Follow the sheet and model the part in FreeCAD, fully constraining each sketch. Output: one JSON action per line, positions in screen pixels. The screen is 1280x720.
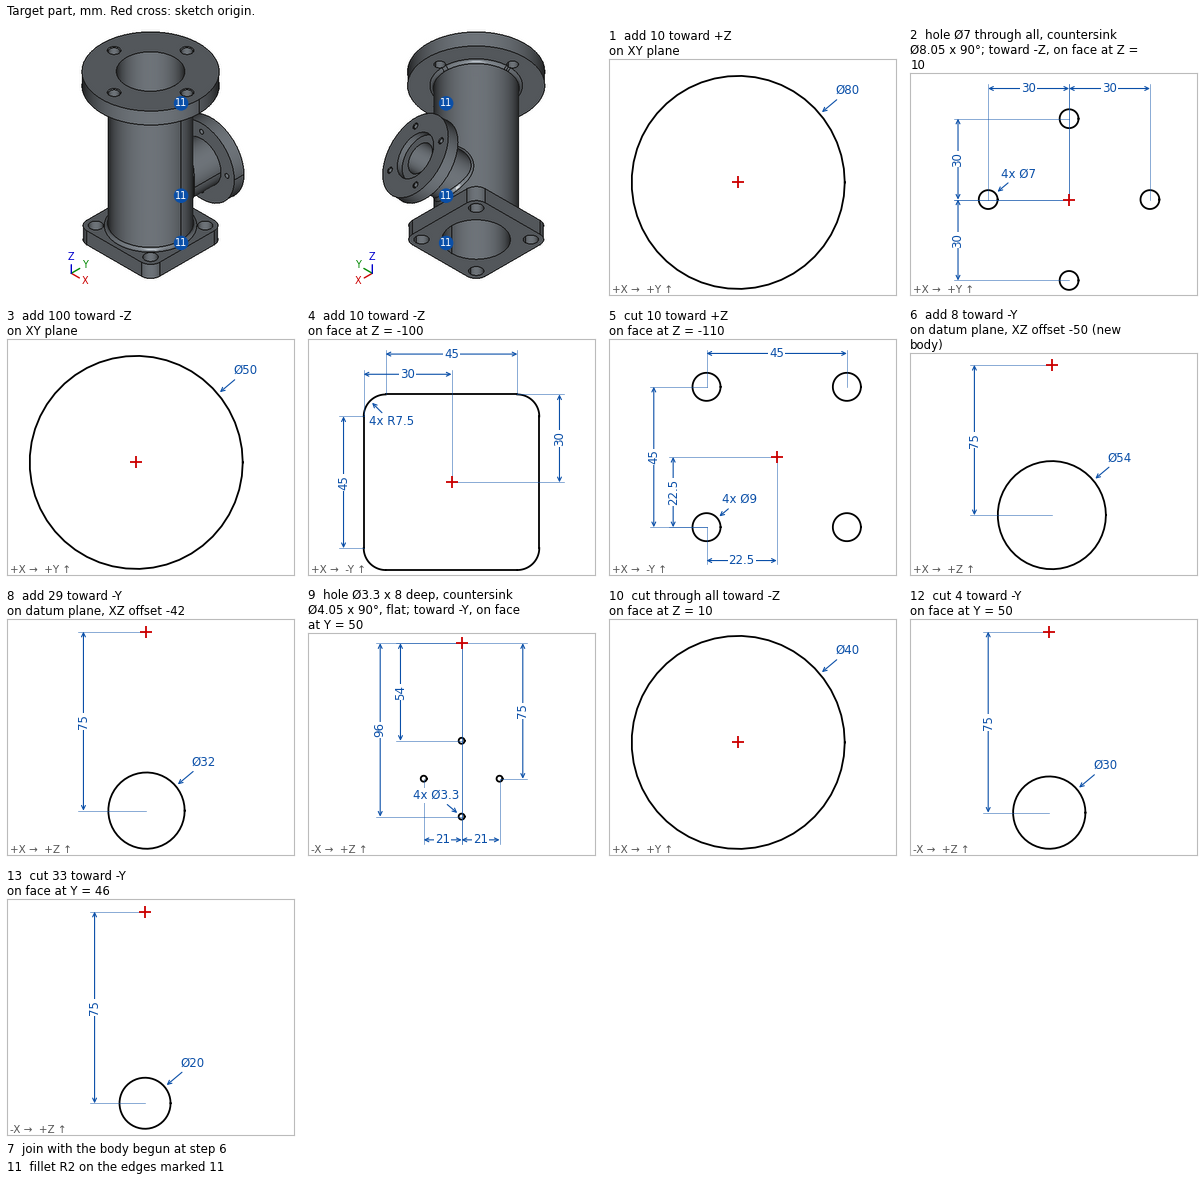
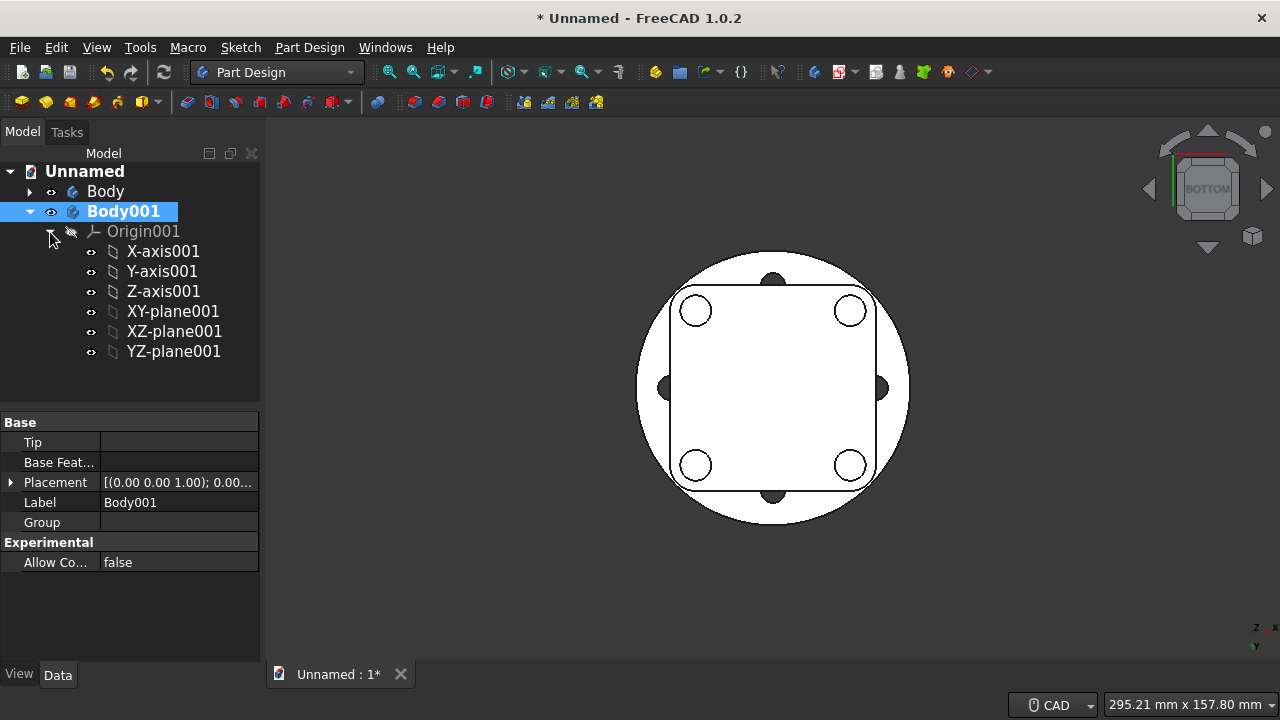
{"action": "left_click", "coordinate": [136, 332]}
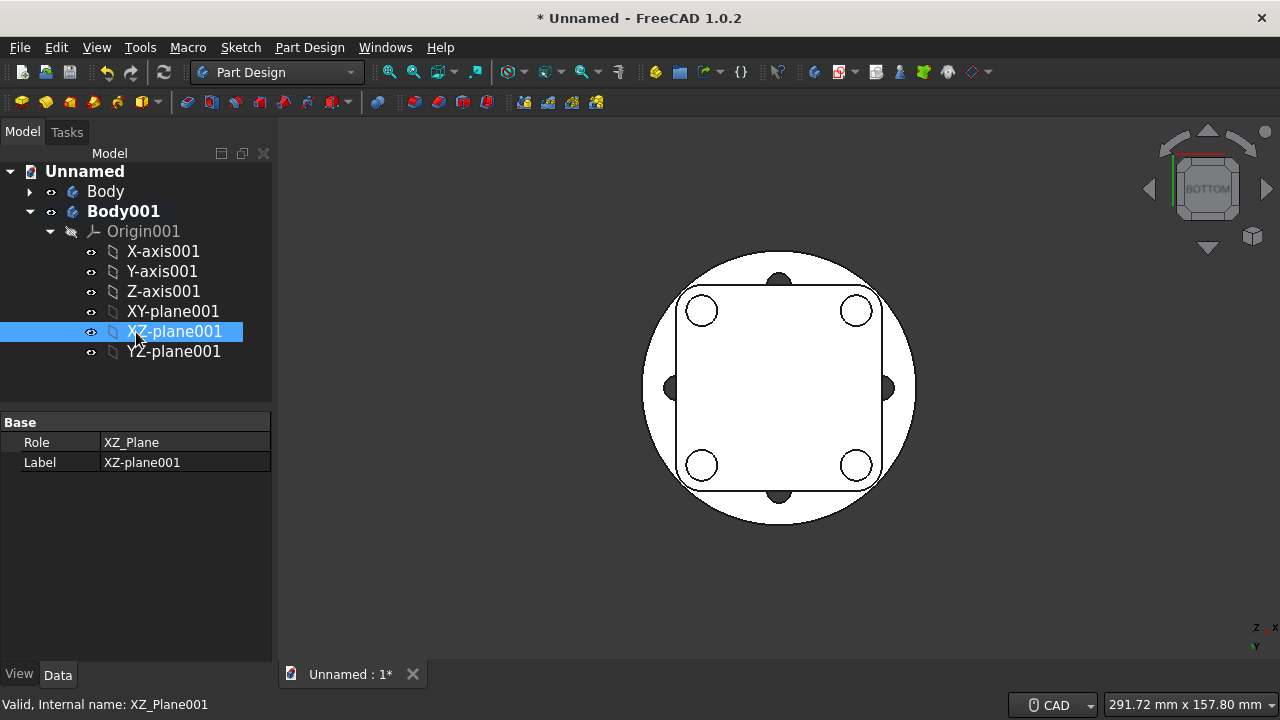
{"action": "left_click", "coordinate": [972, 72]}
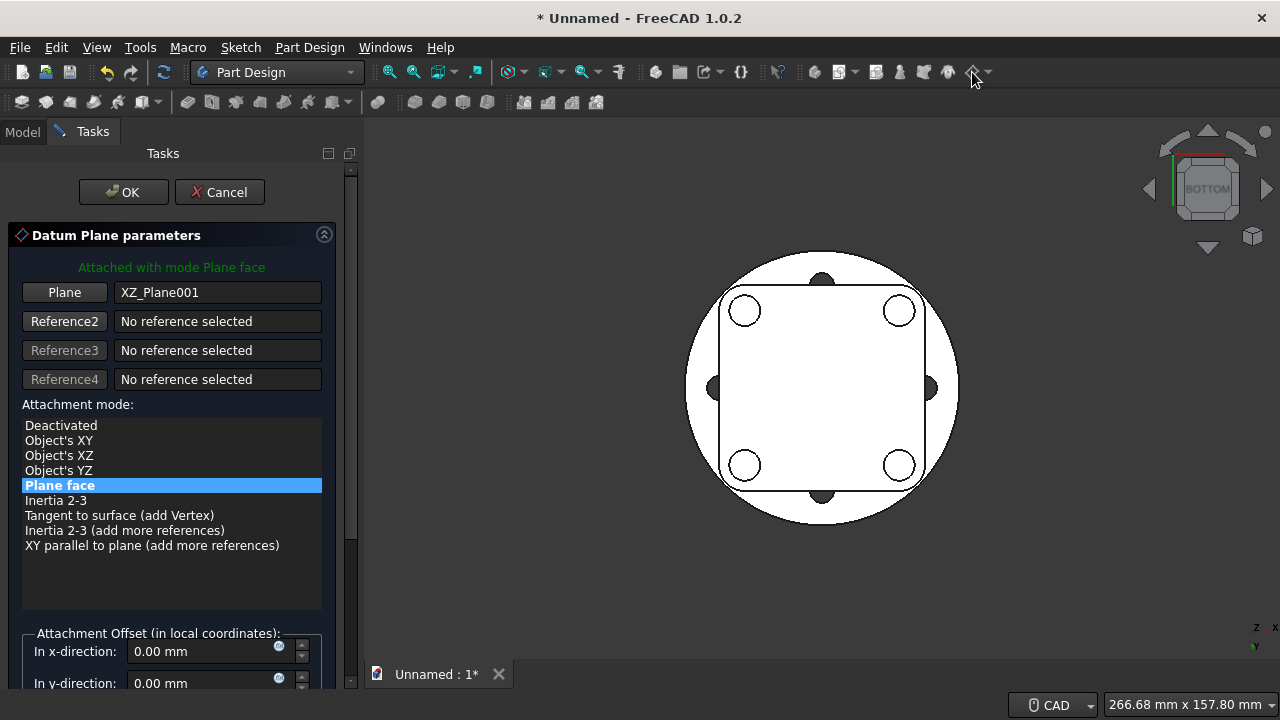
{"action": "scroll", "coordinate": [351, 426], "scroll_direction": "down", "scroll_amount": 2}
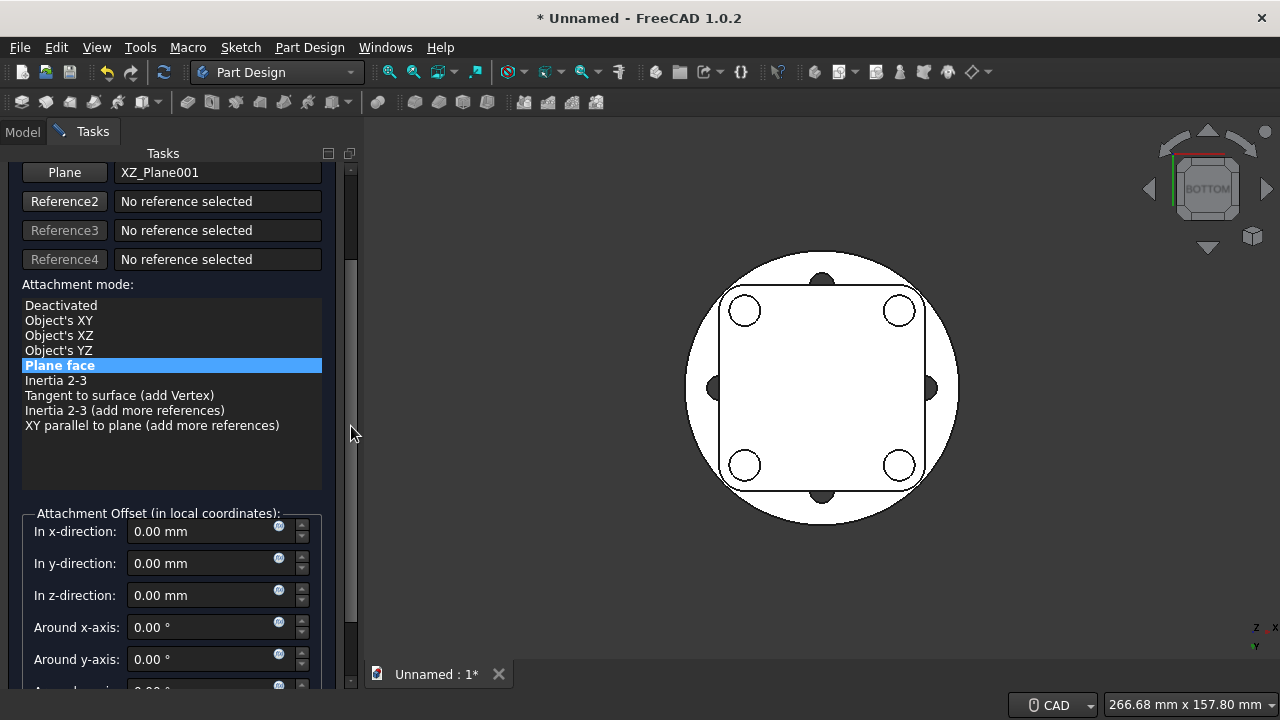
{"action": "triple_click", "coordinate": [210, 595]}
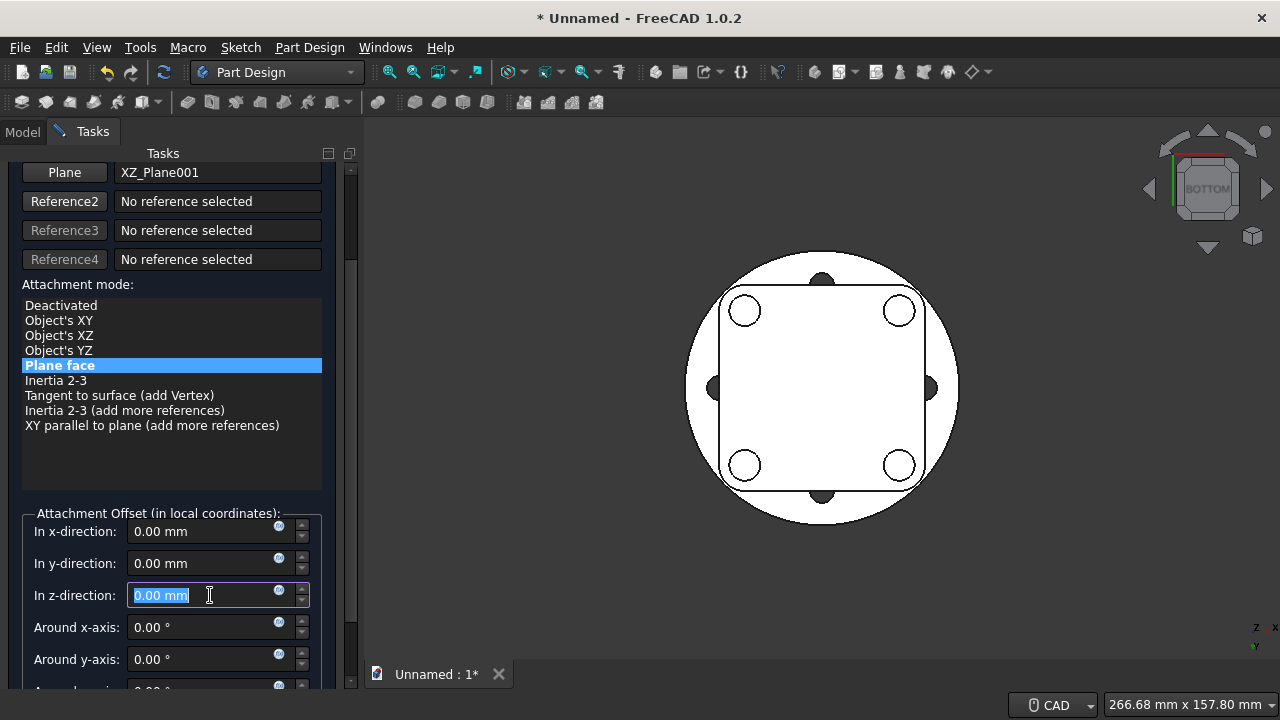
{"action": "type", "text": "-50"}
{"action": "key", "text": "Tab"}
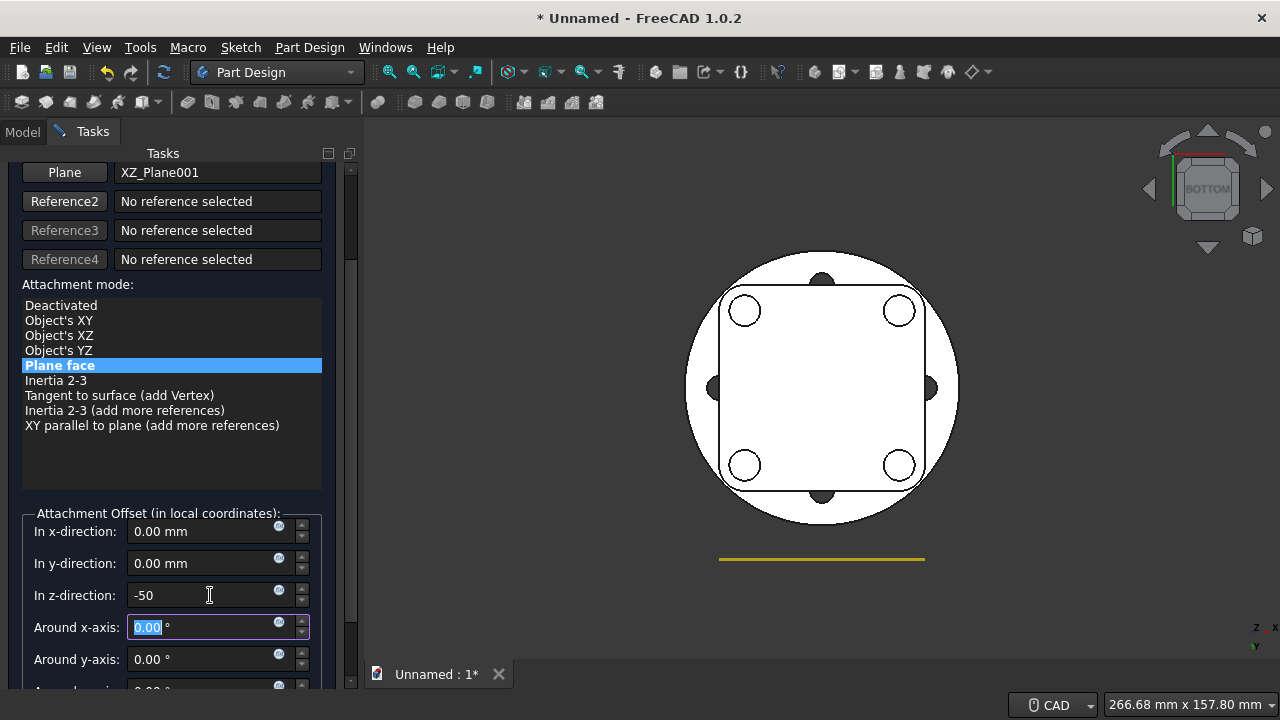
{"action": "scroll", "coordinate": [351, 426], "scroll_direction": "up", "scroll_amount": 3}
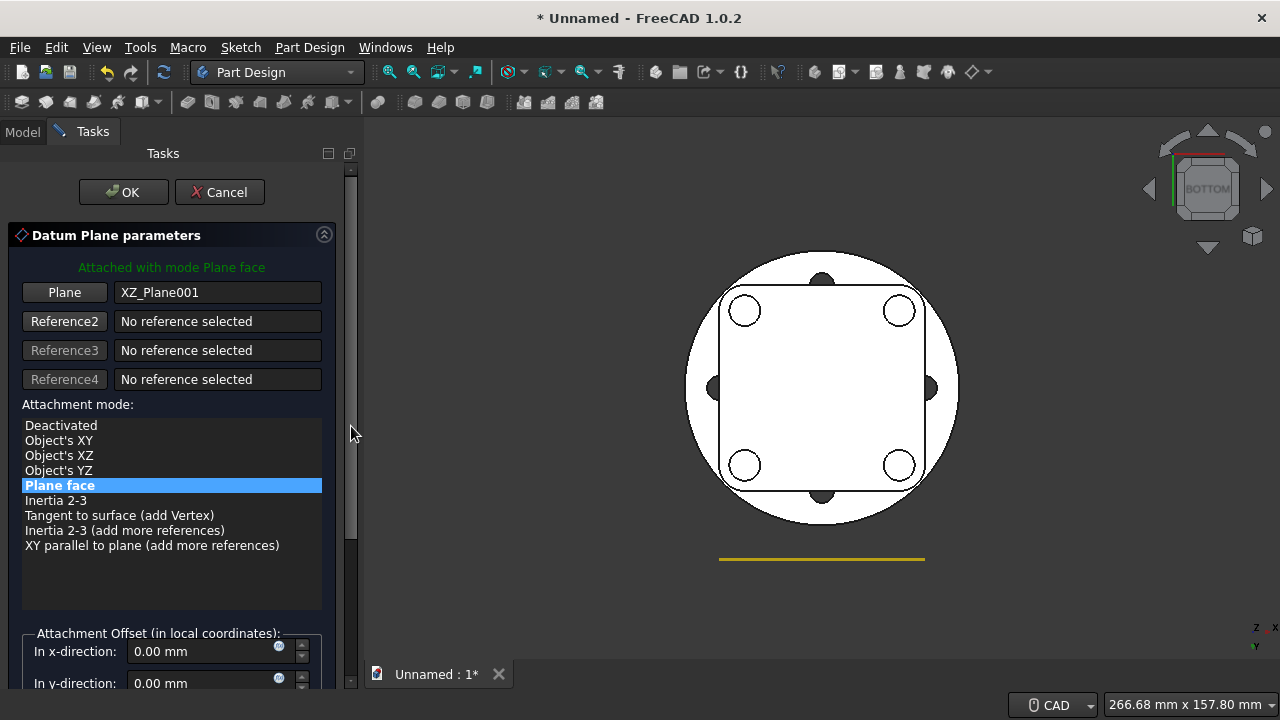
{"action": "left_click", "coordinate": [124, 192]}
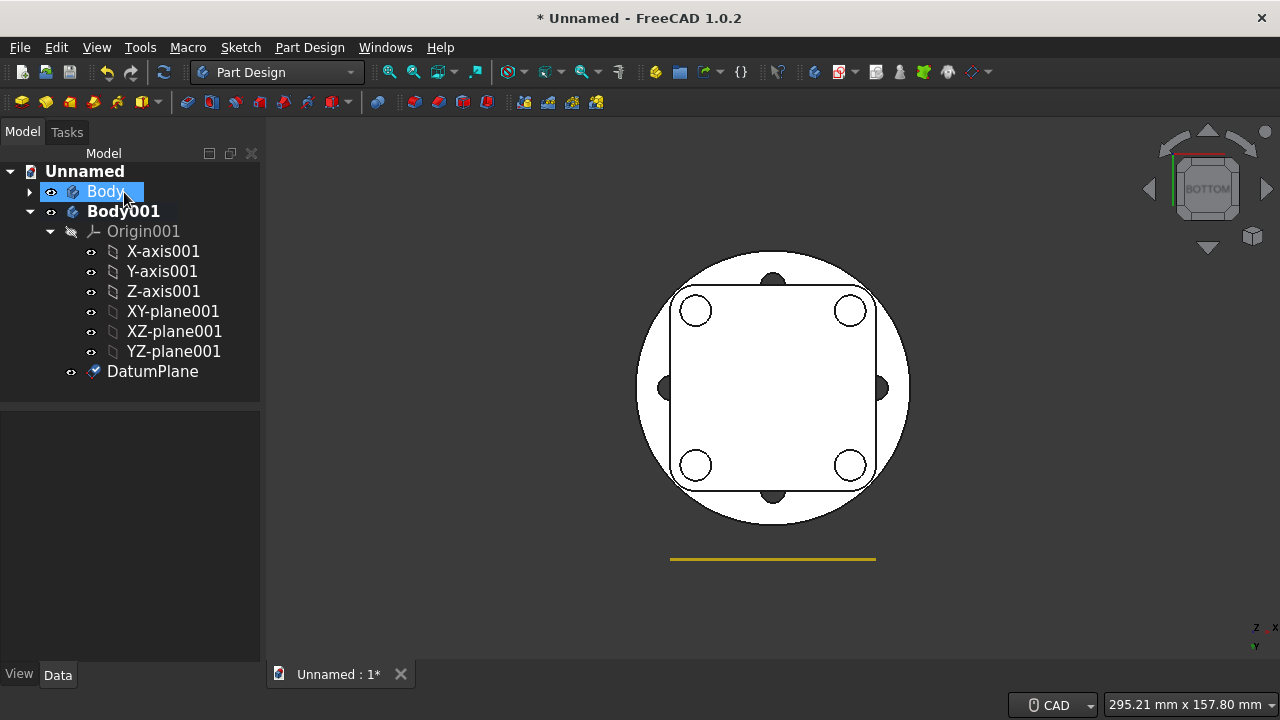
{"action": "left_click", "coordinate": [116, 372]}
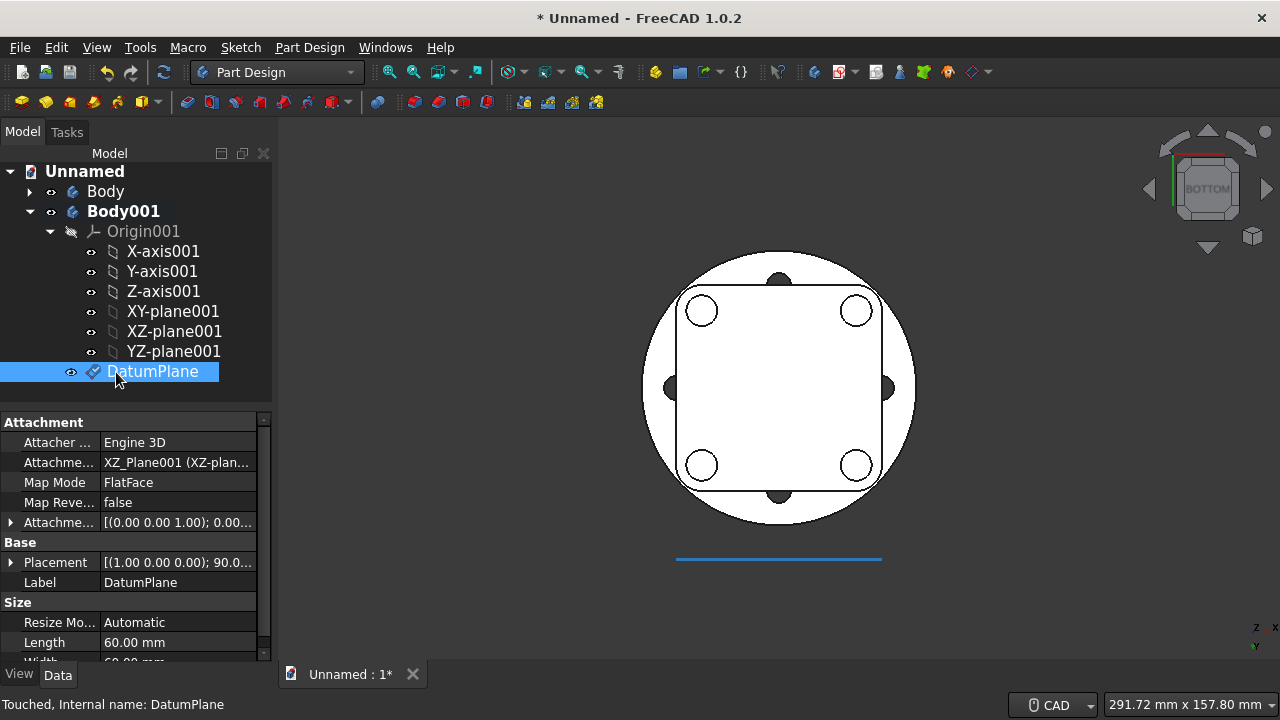
{"action": "left_click", "coordinate": [840, 72]}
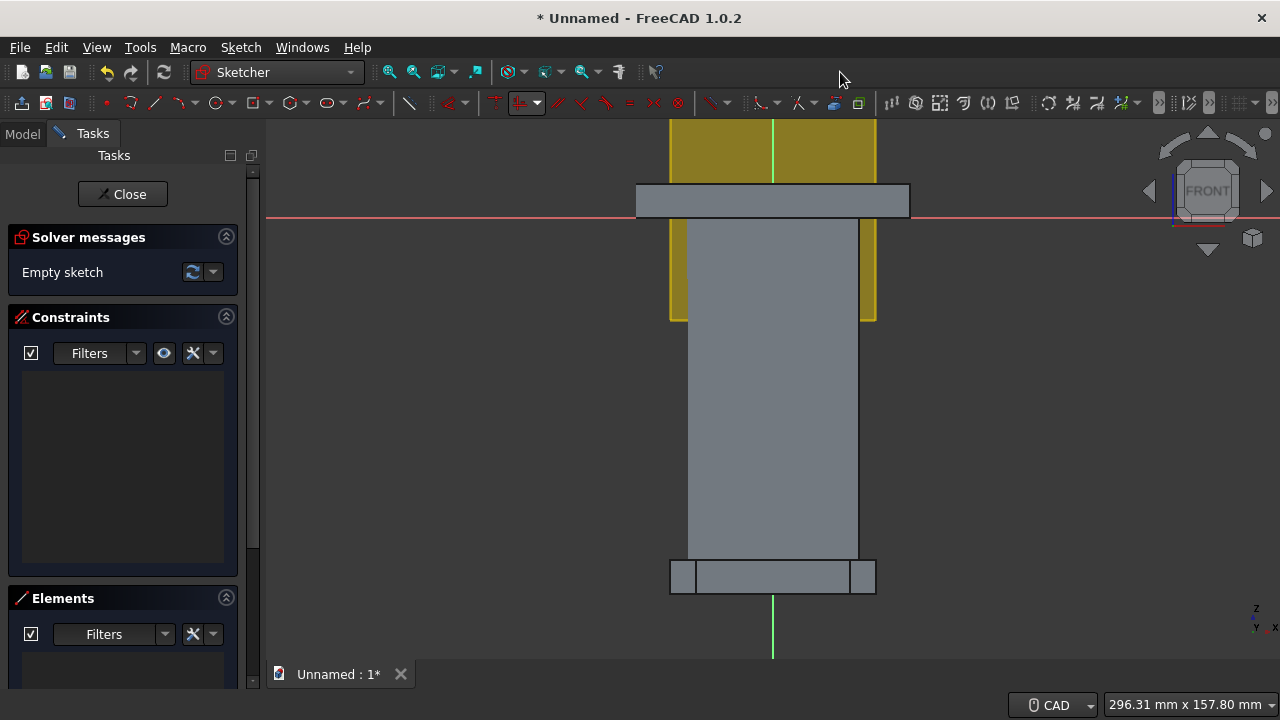
{"action": "left_click", "coordinate": [216, 104]}